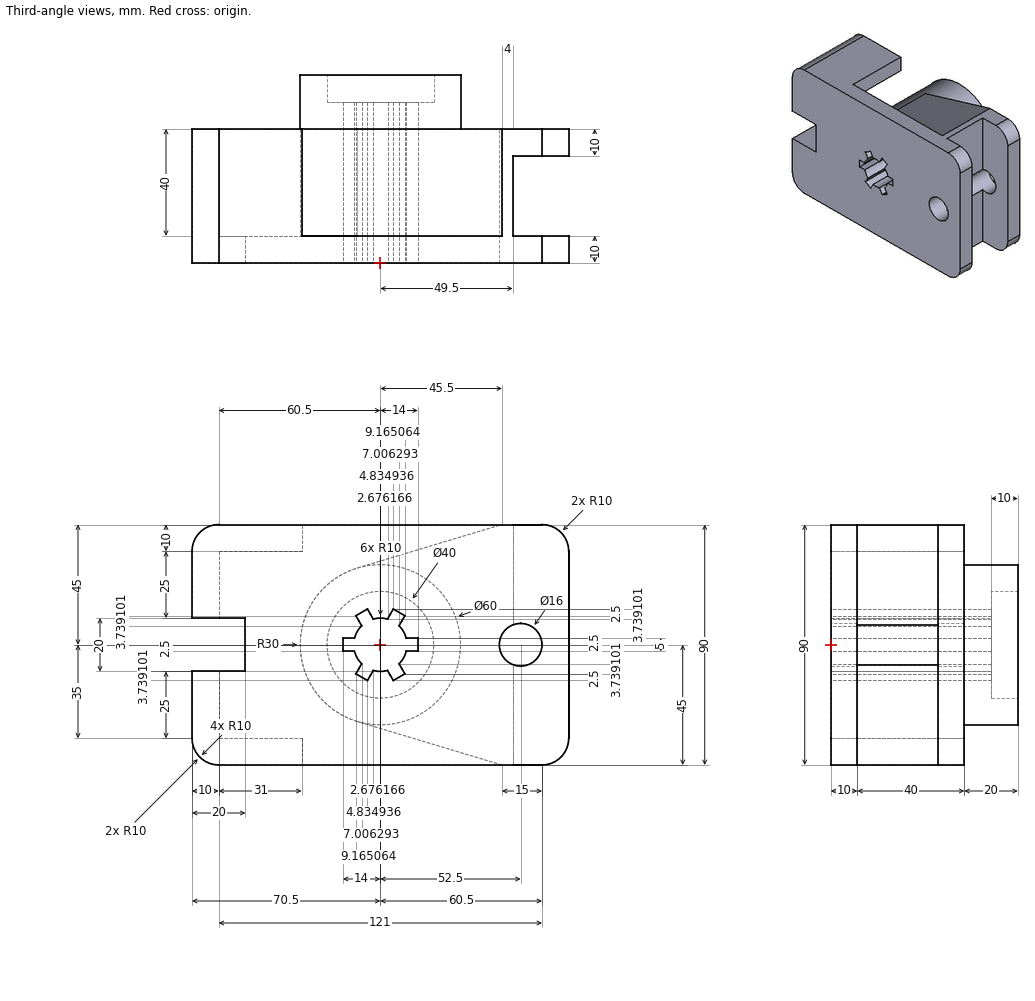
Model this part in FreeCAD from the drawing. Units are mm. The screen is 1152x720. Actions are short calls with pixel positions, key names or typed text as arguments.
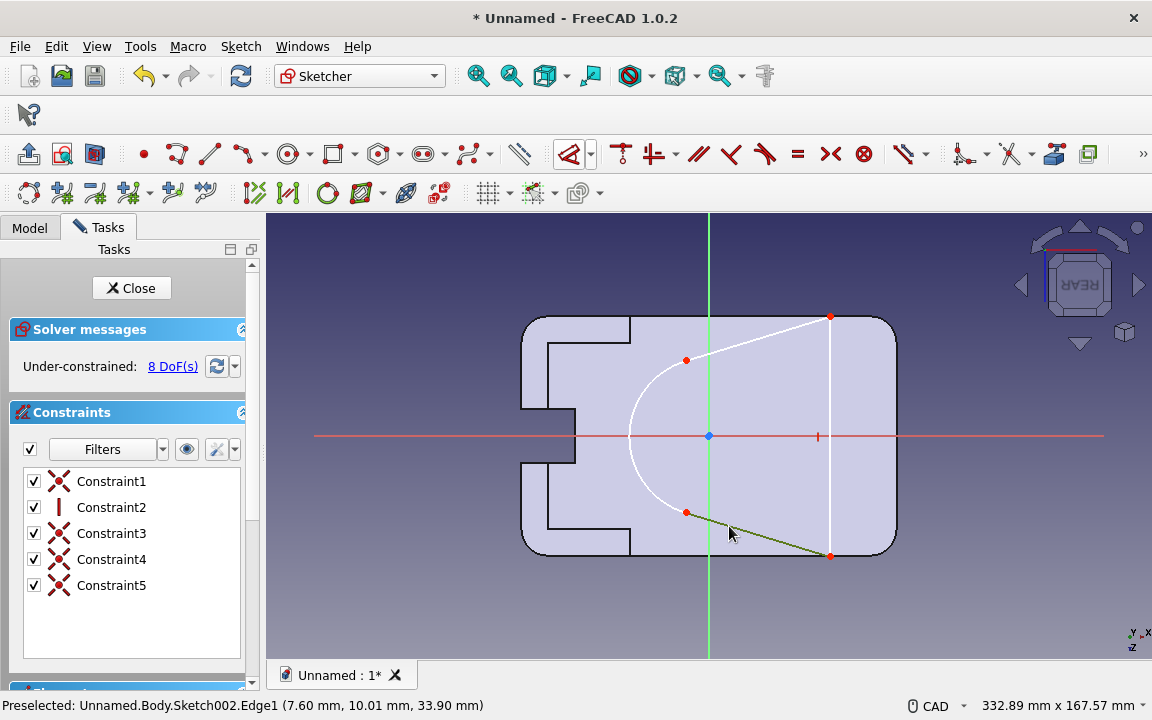
click(640, 398)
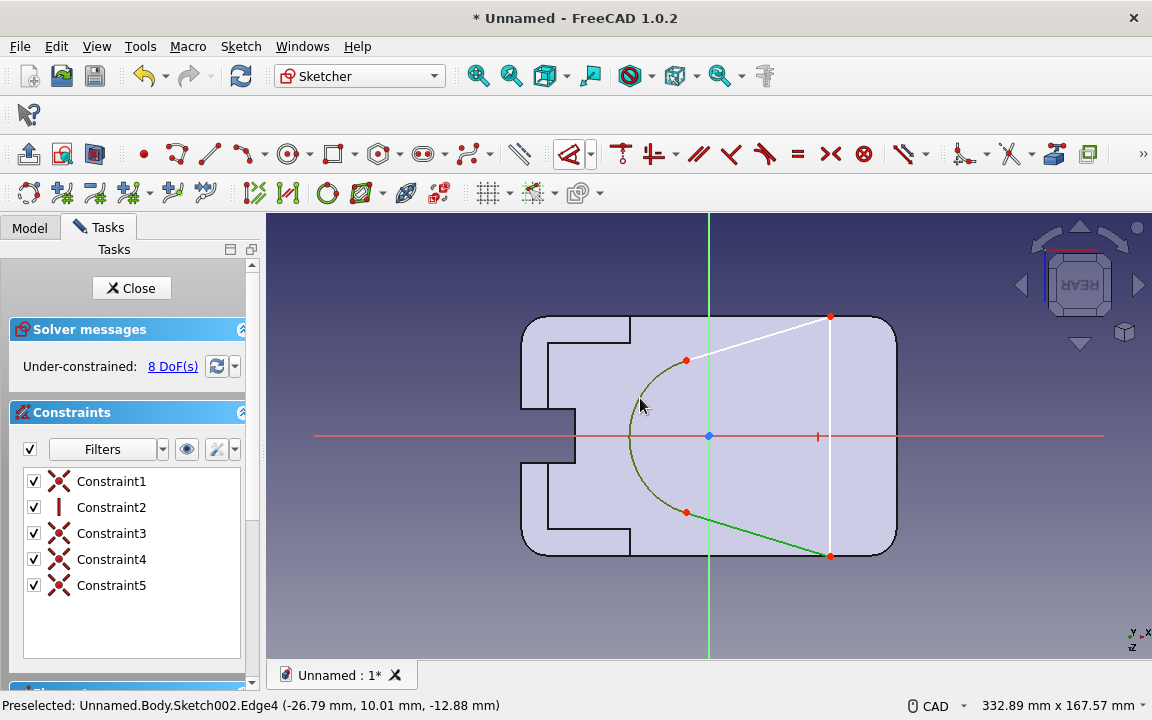
click(765, 154)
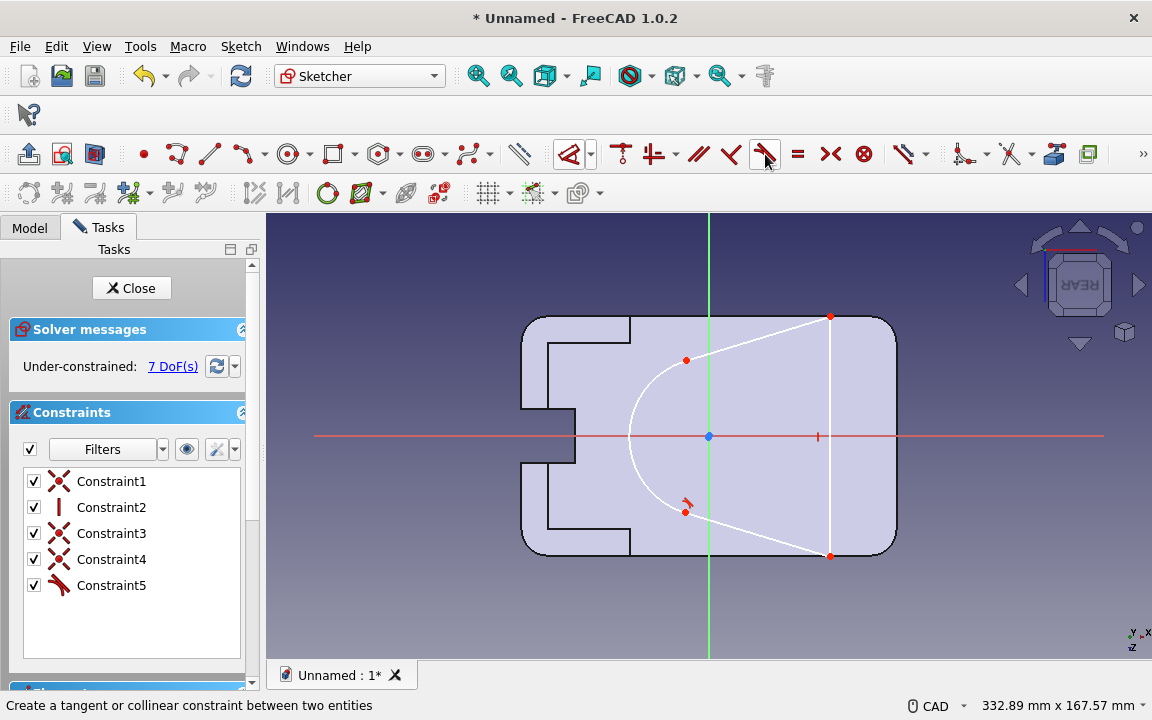
click(787, 330)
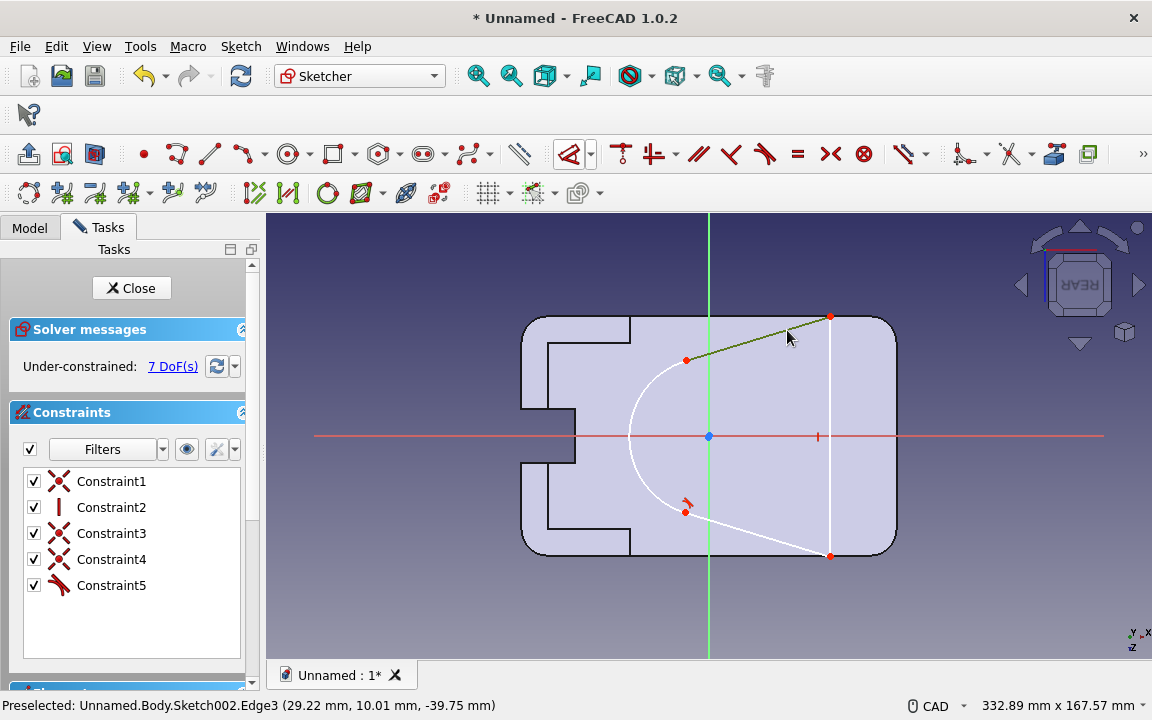
click(640, 398)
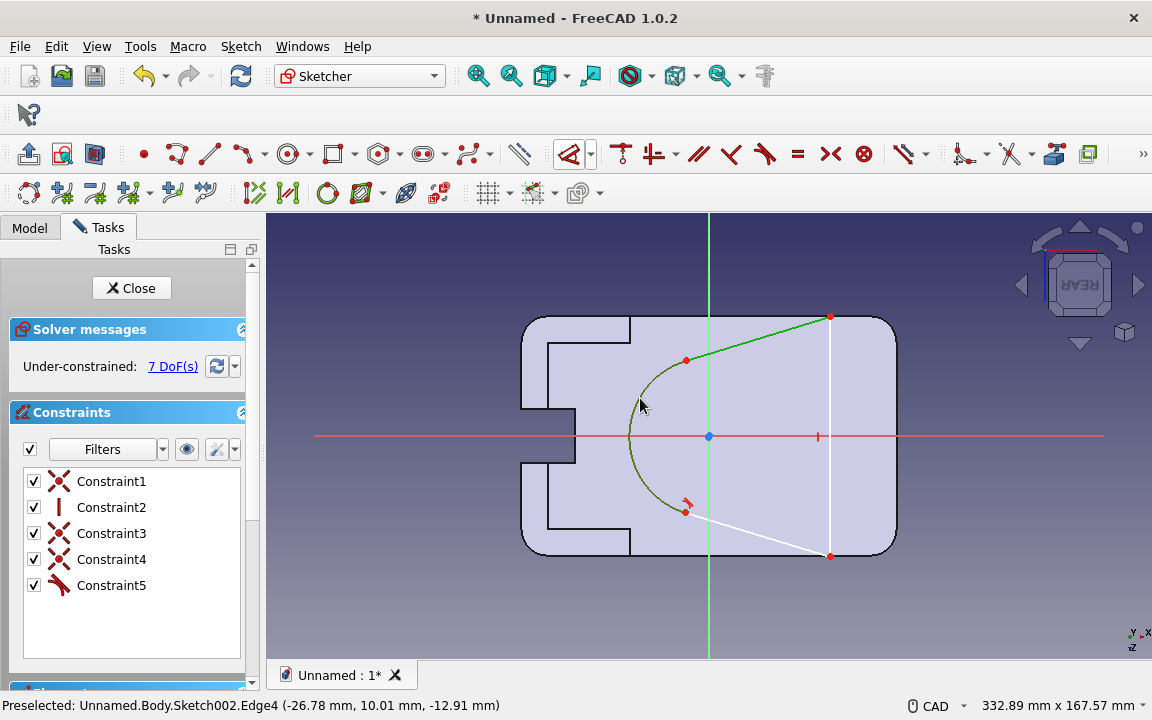
click(765, 154)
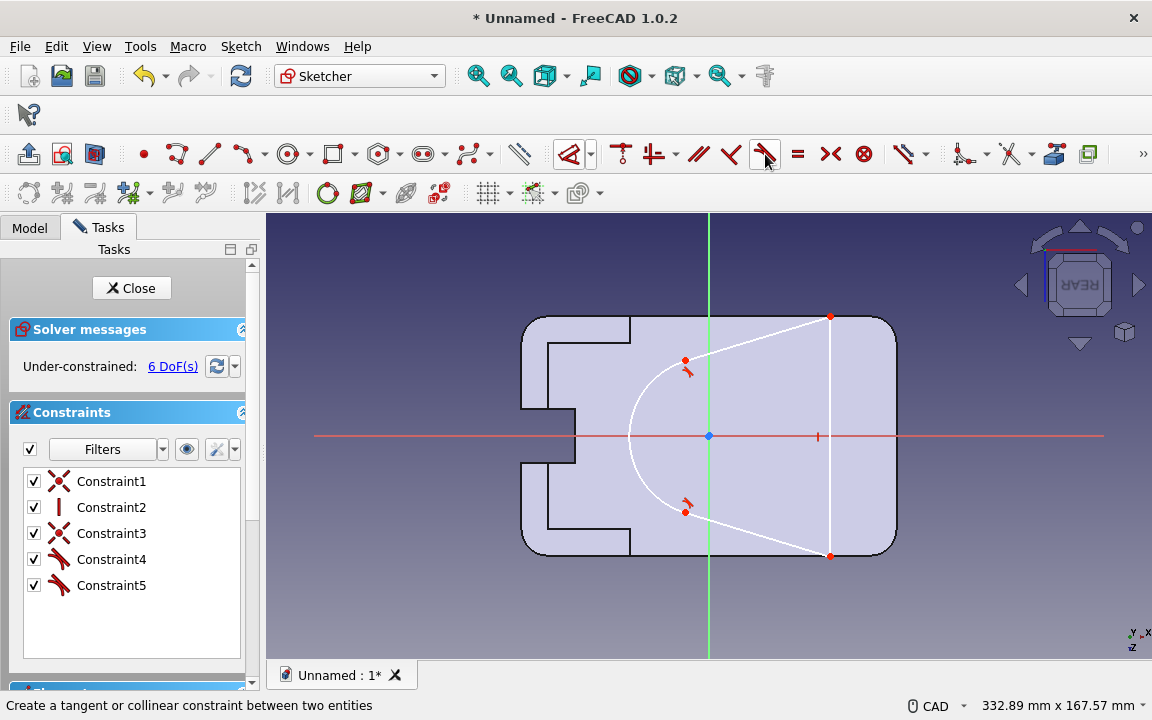
drag(699, 426, 719, 447)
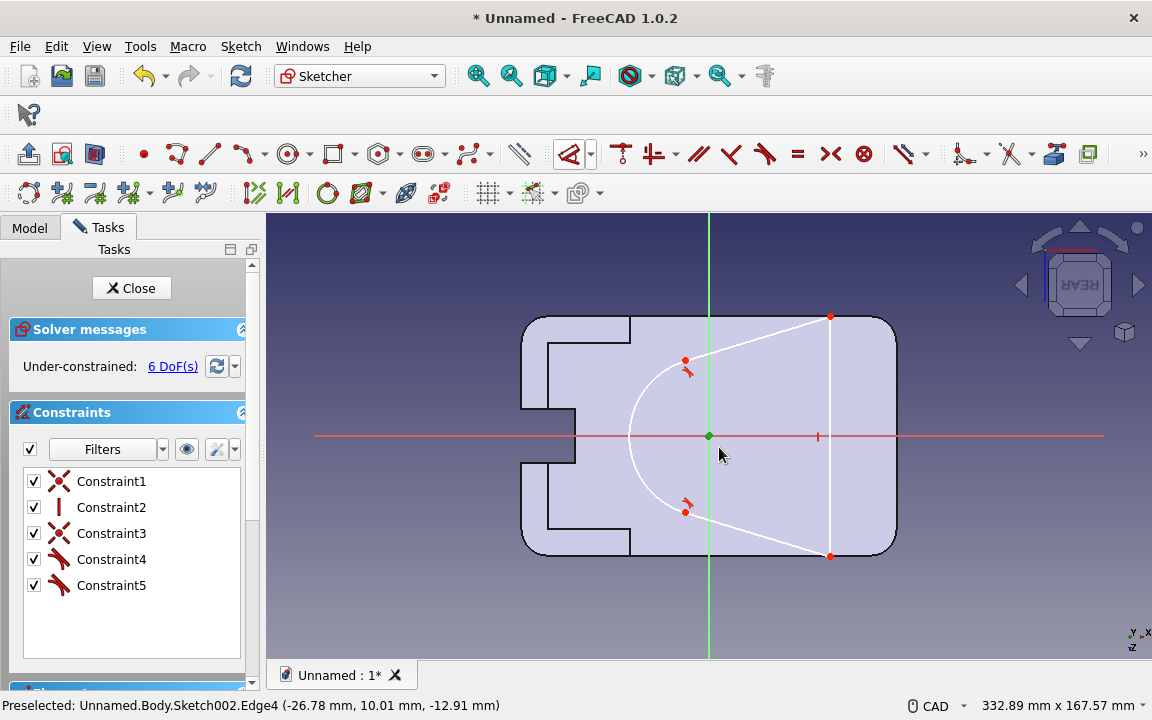
click(621, 154)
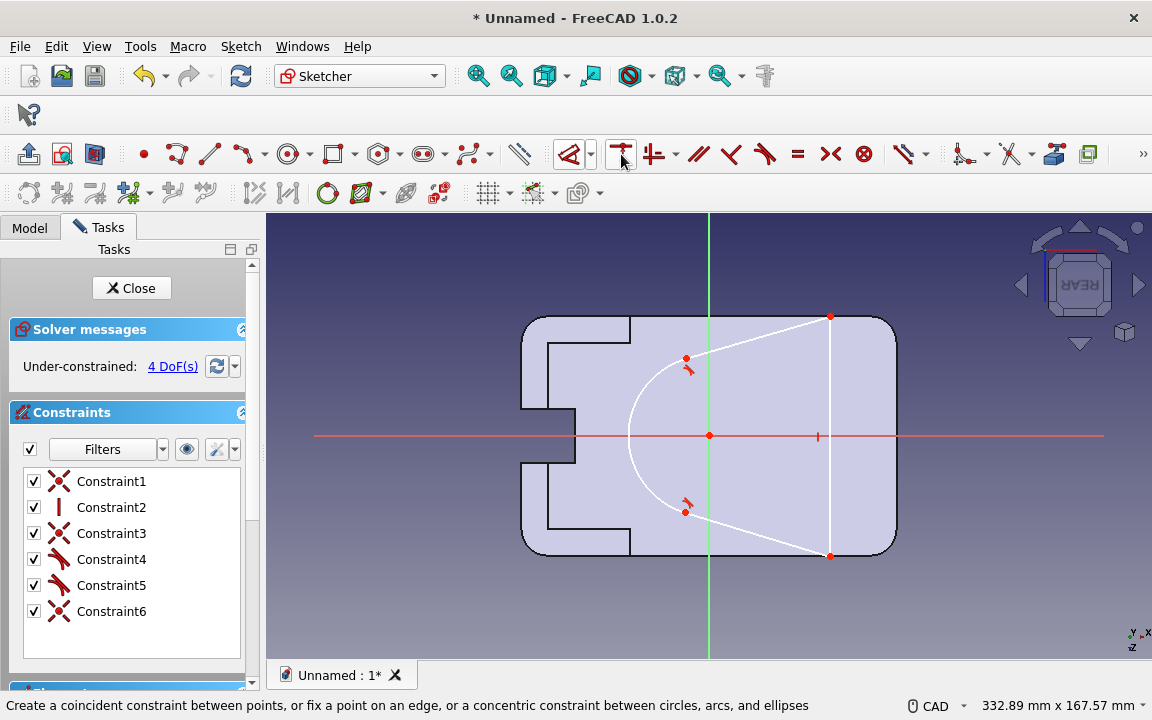
click(639, 396)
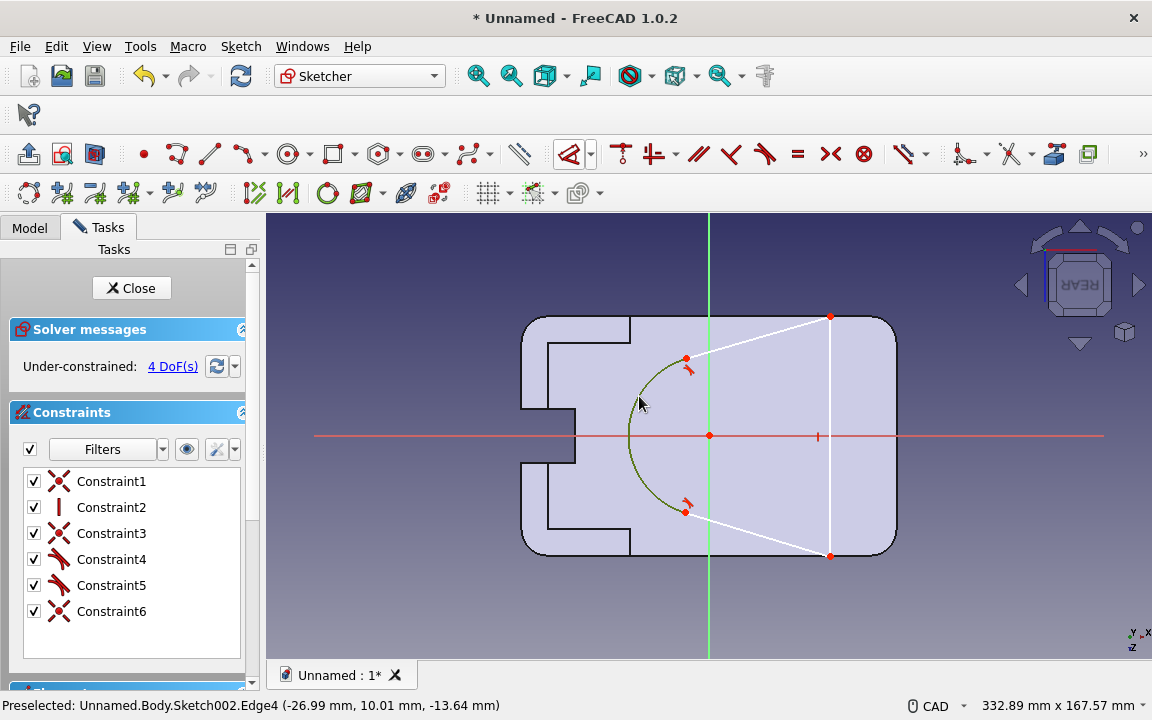
click(590, 154)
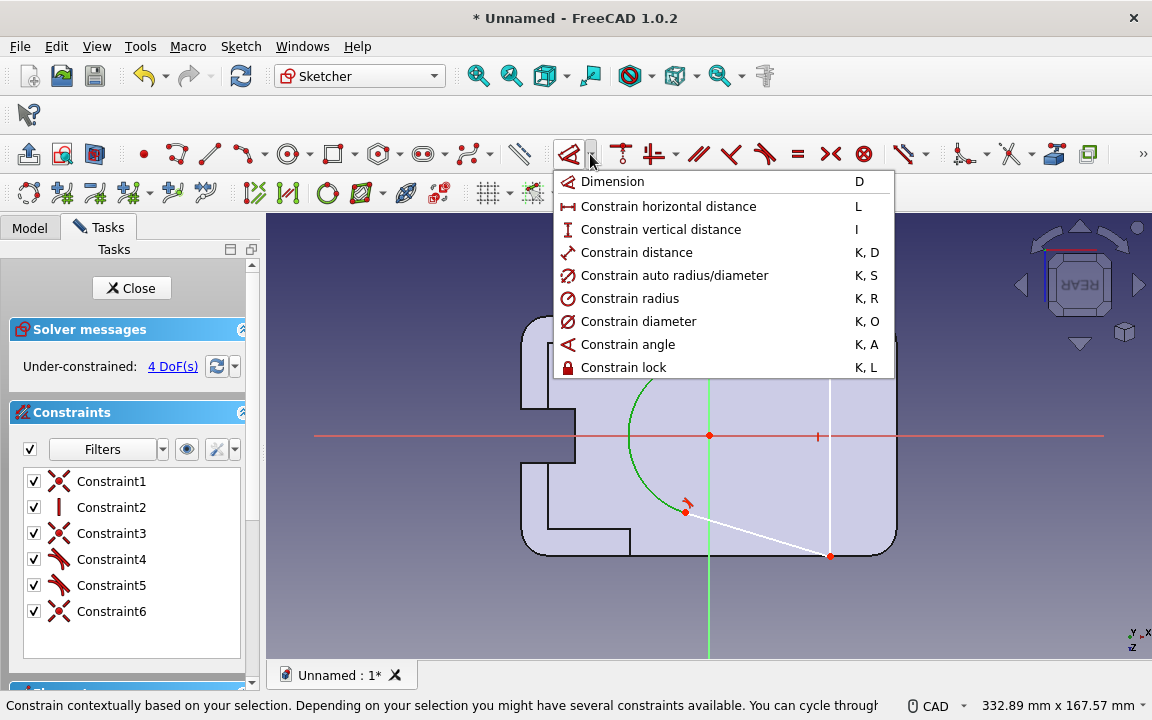
click(724, 298)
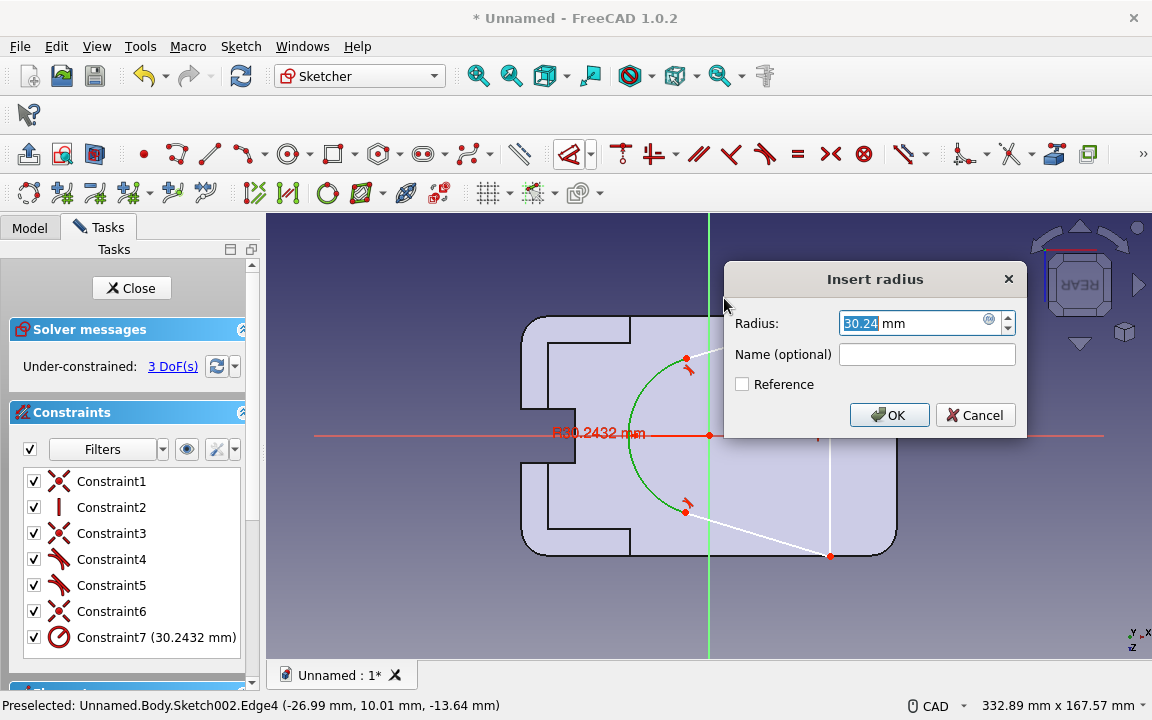
text(30)
key(Return)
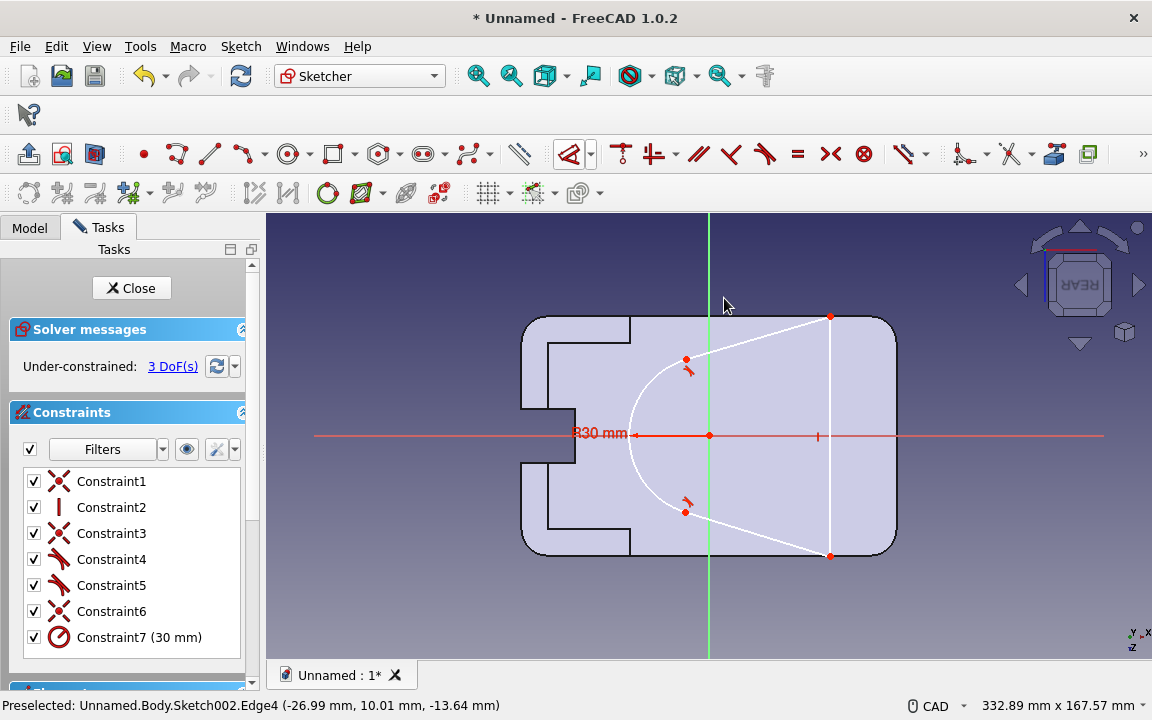
click(830, 485)